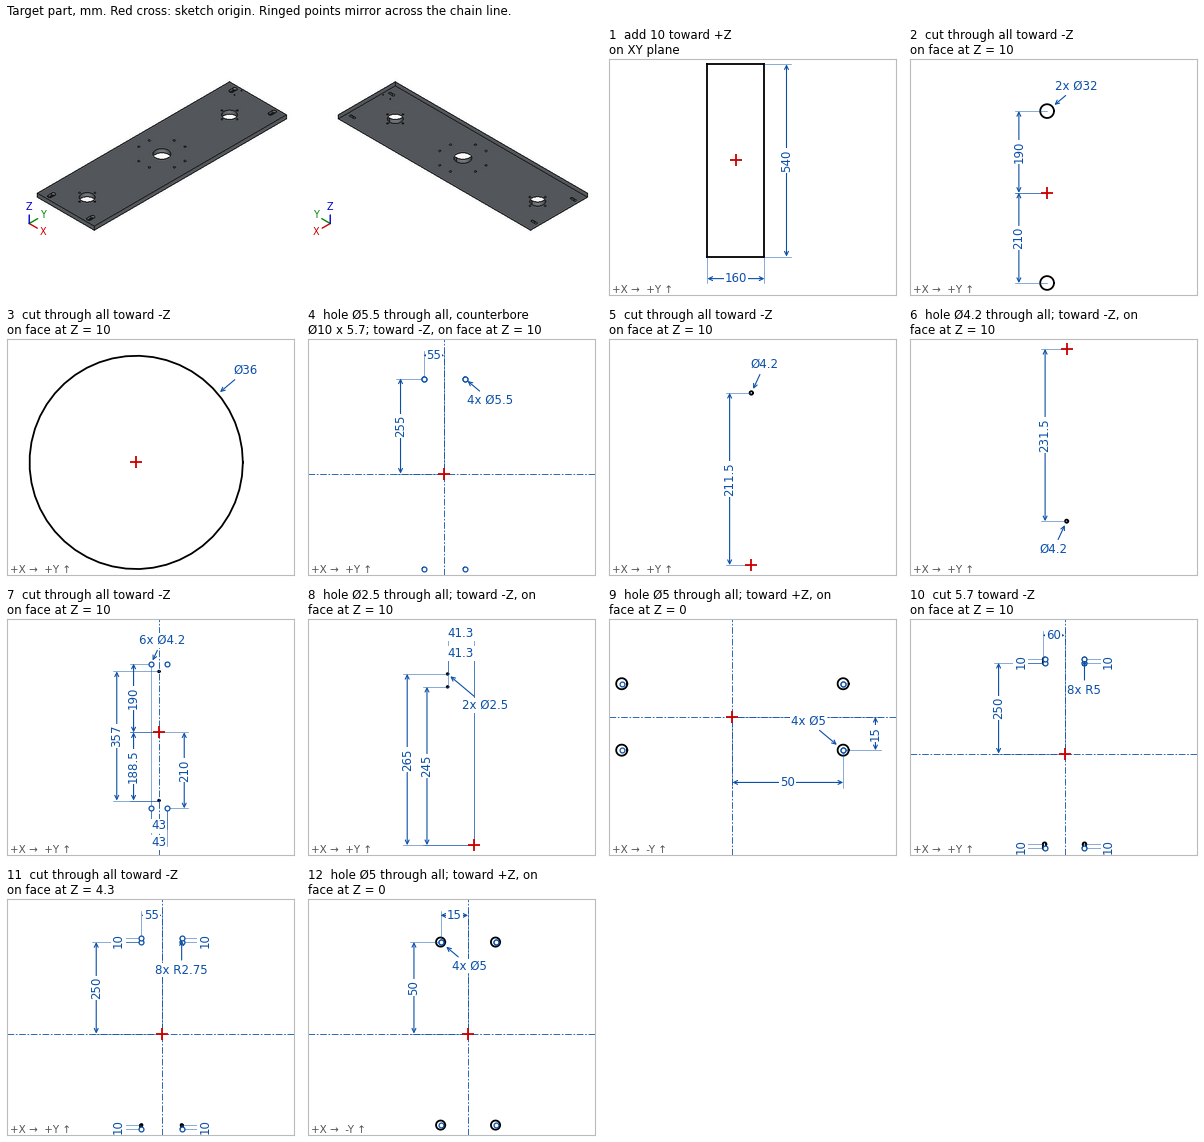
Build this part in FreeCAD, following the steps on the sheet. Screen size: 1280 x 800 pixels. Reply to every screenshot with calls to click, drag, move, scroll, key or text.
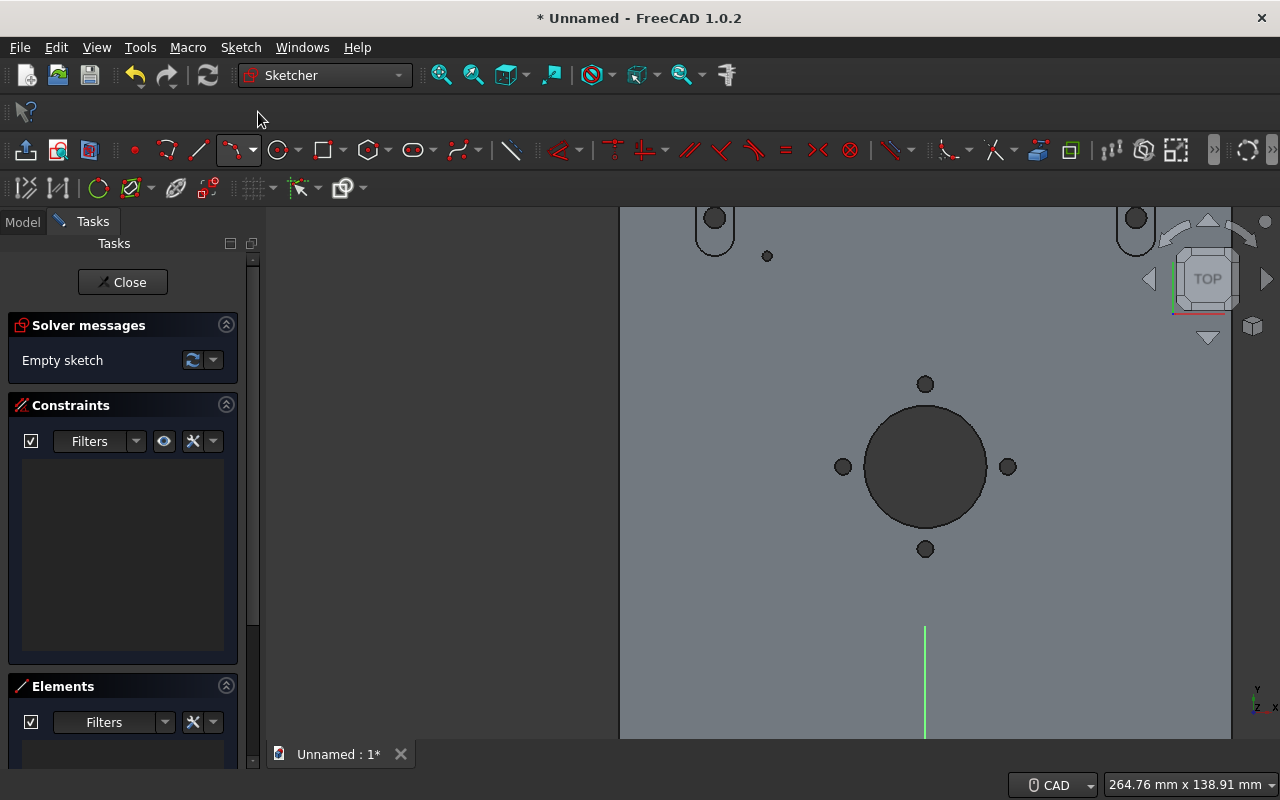
scroll(661, 330, down, 9)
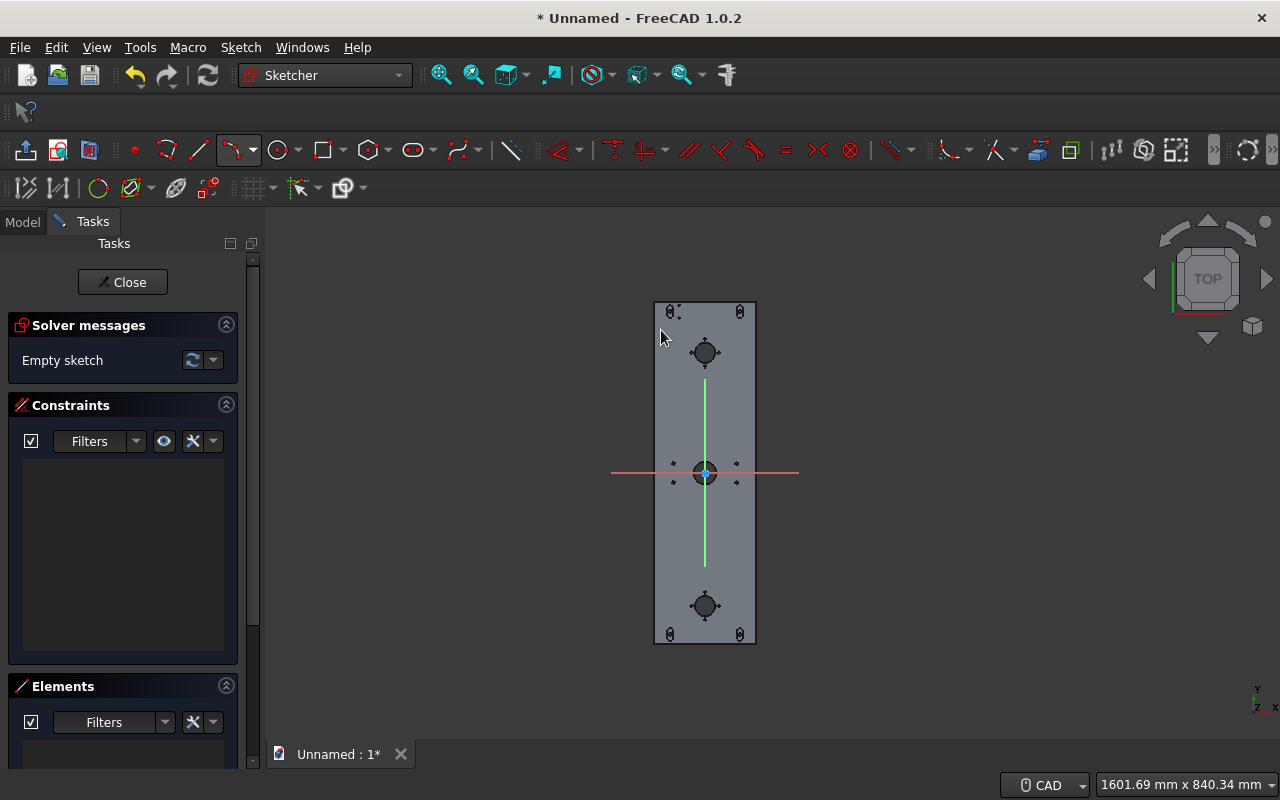
key(g)
key(s)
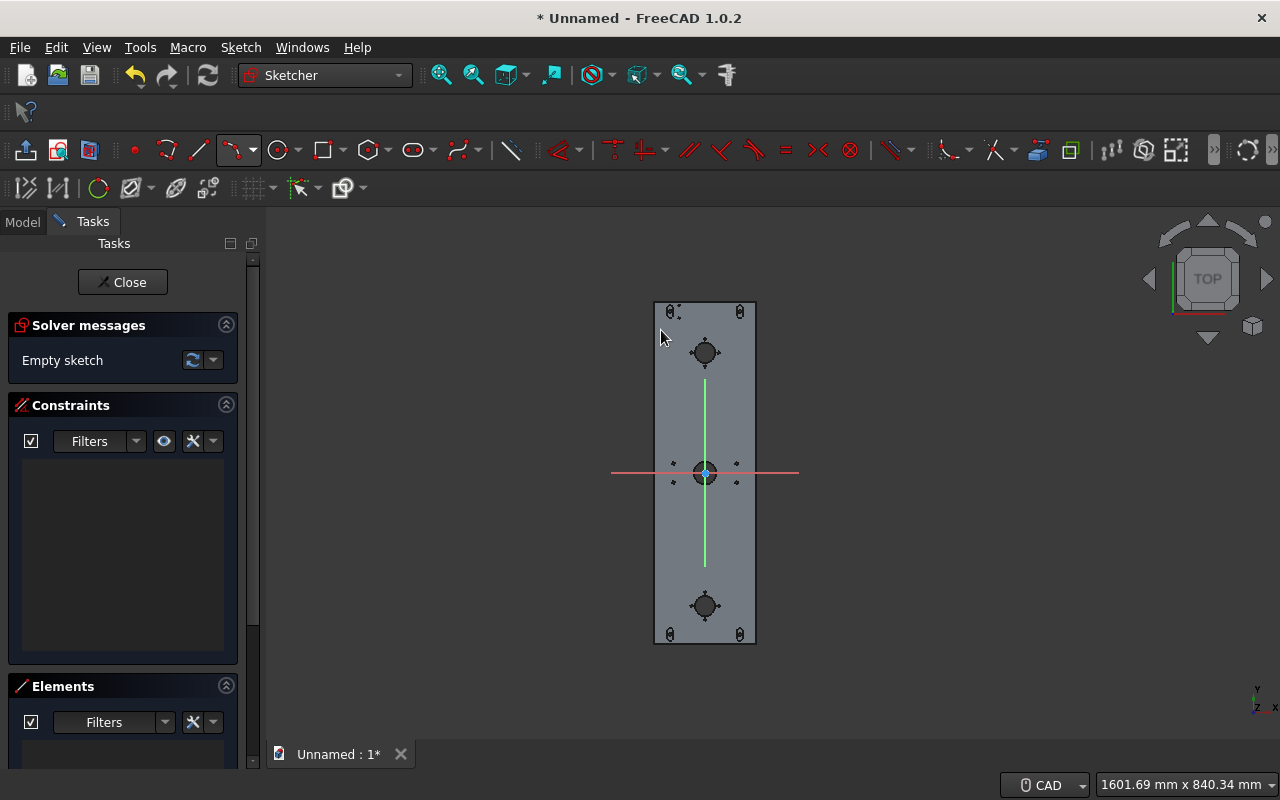
scroll(670, 315, up, 13)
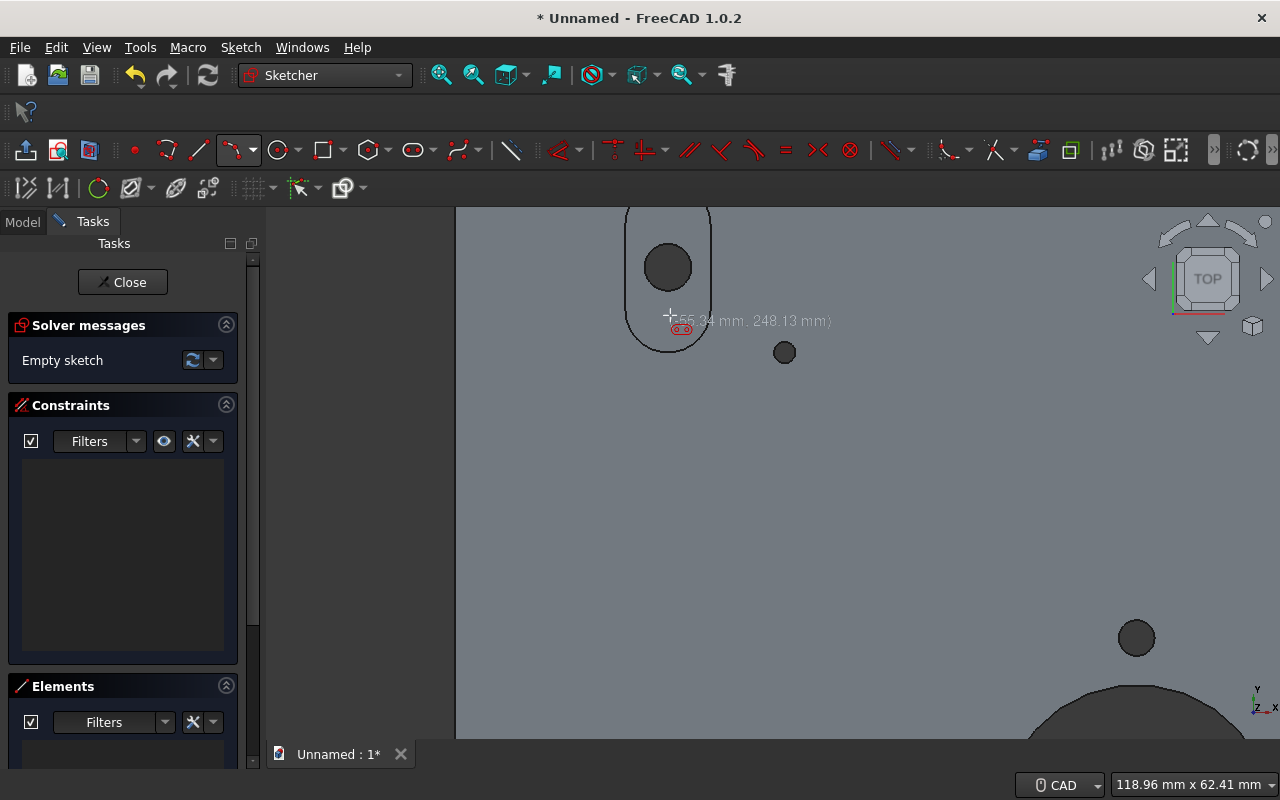
scroll(670, 315, down, 13)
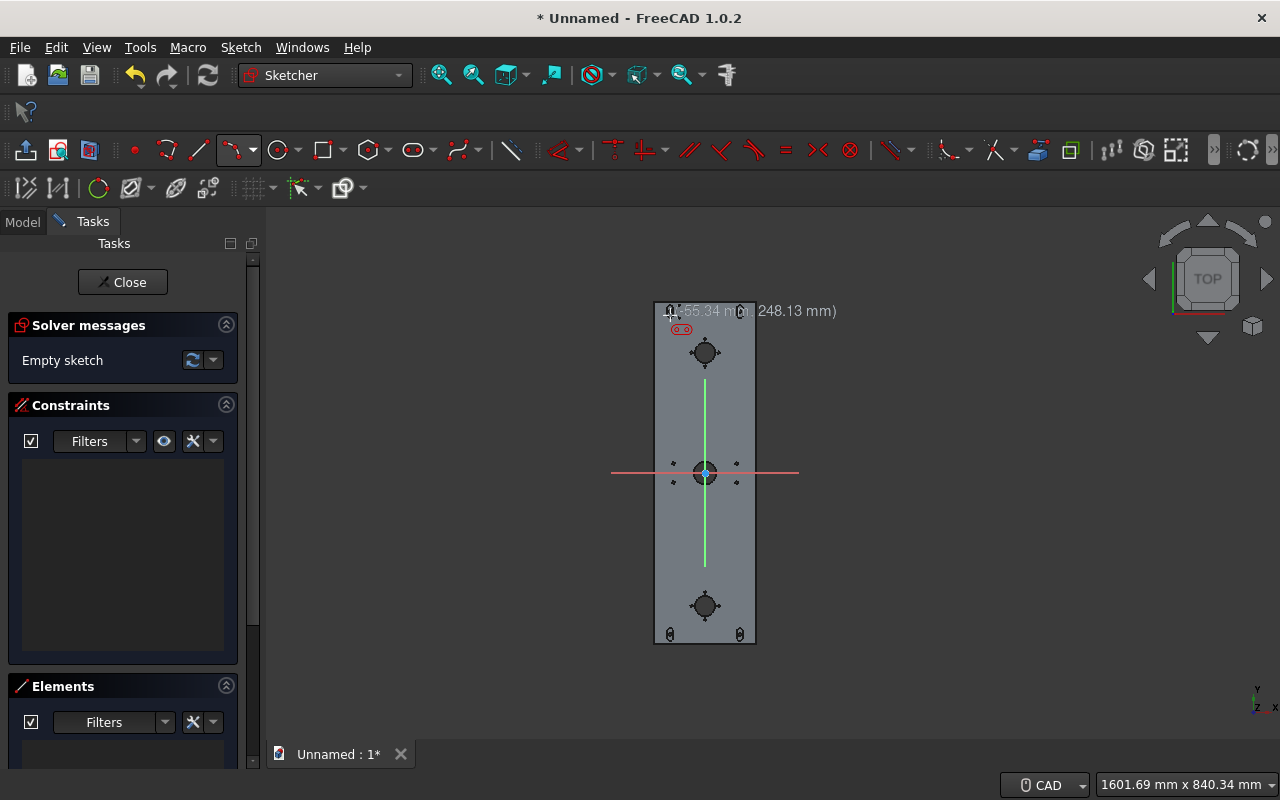
click(670, 315)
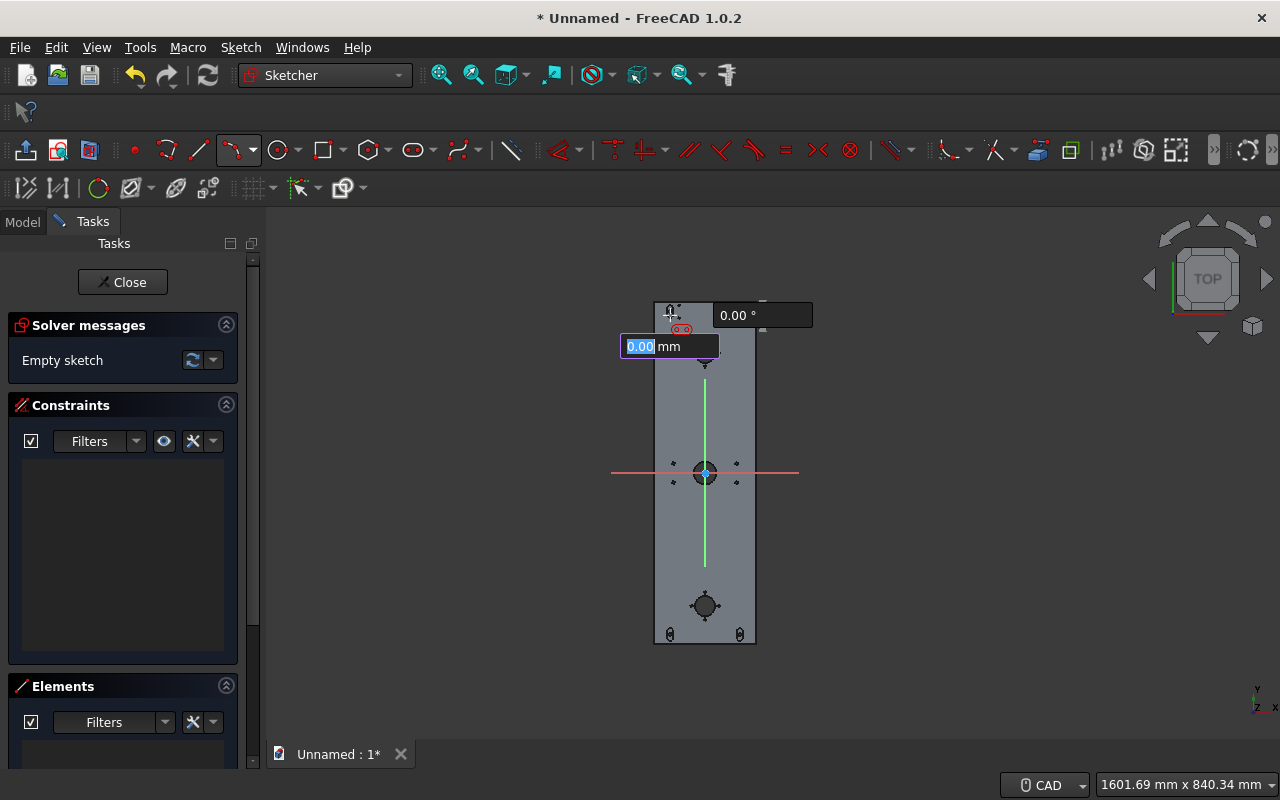
scroll(670, 308, up, 5)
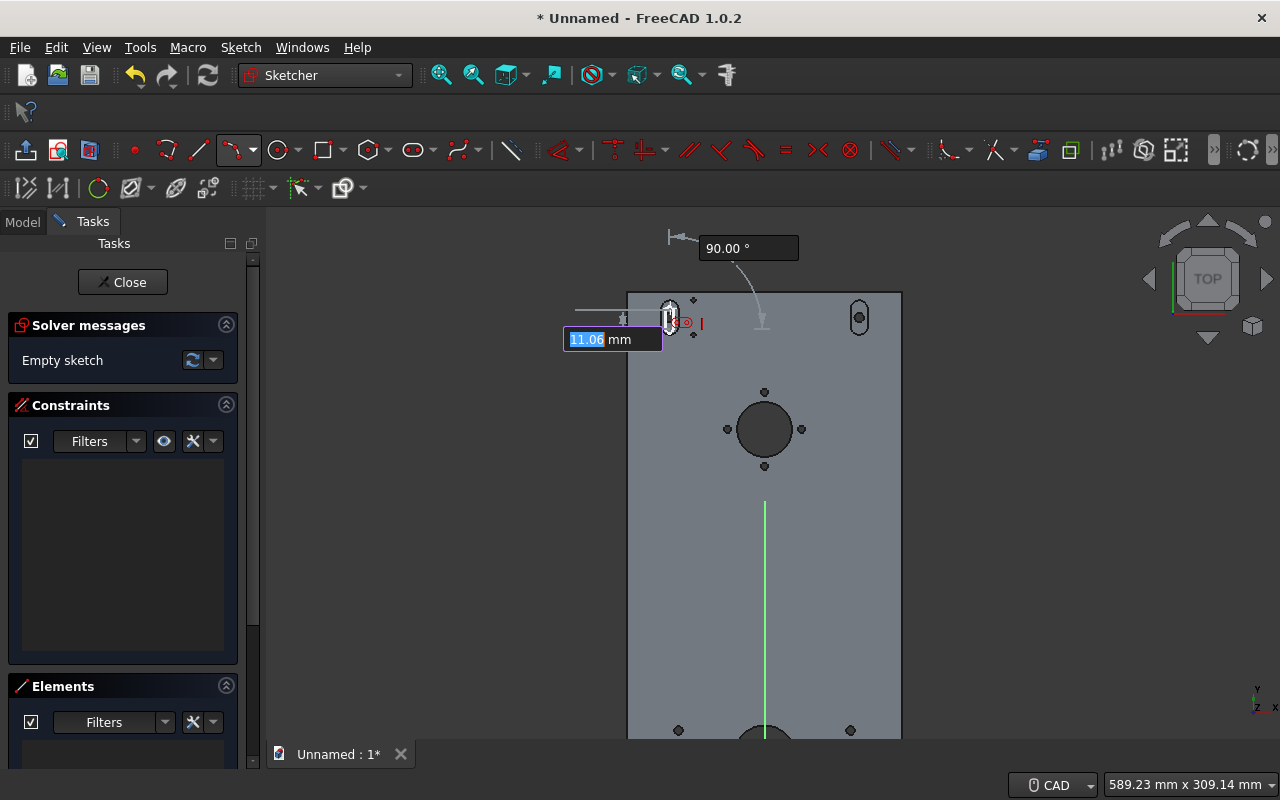
click(669, 309)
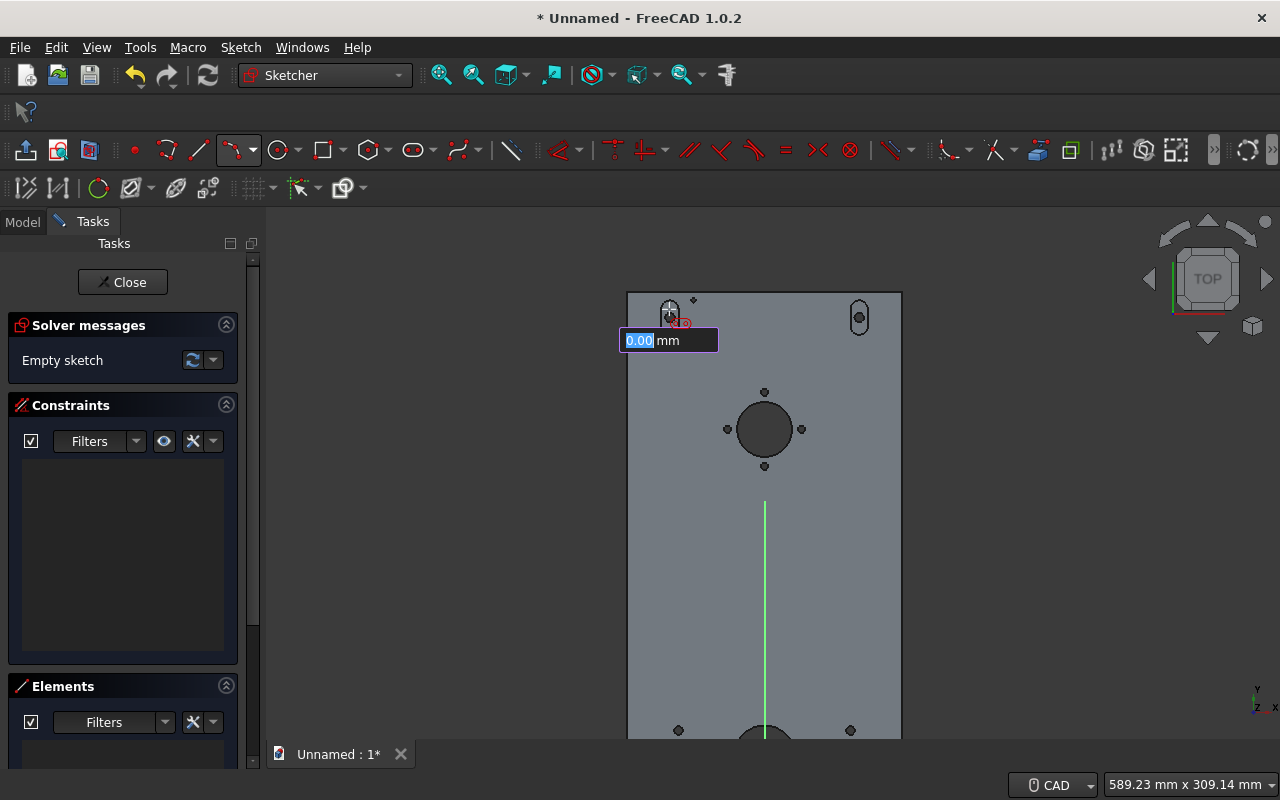
scroll(675, 318, up, 7)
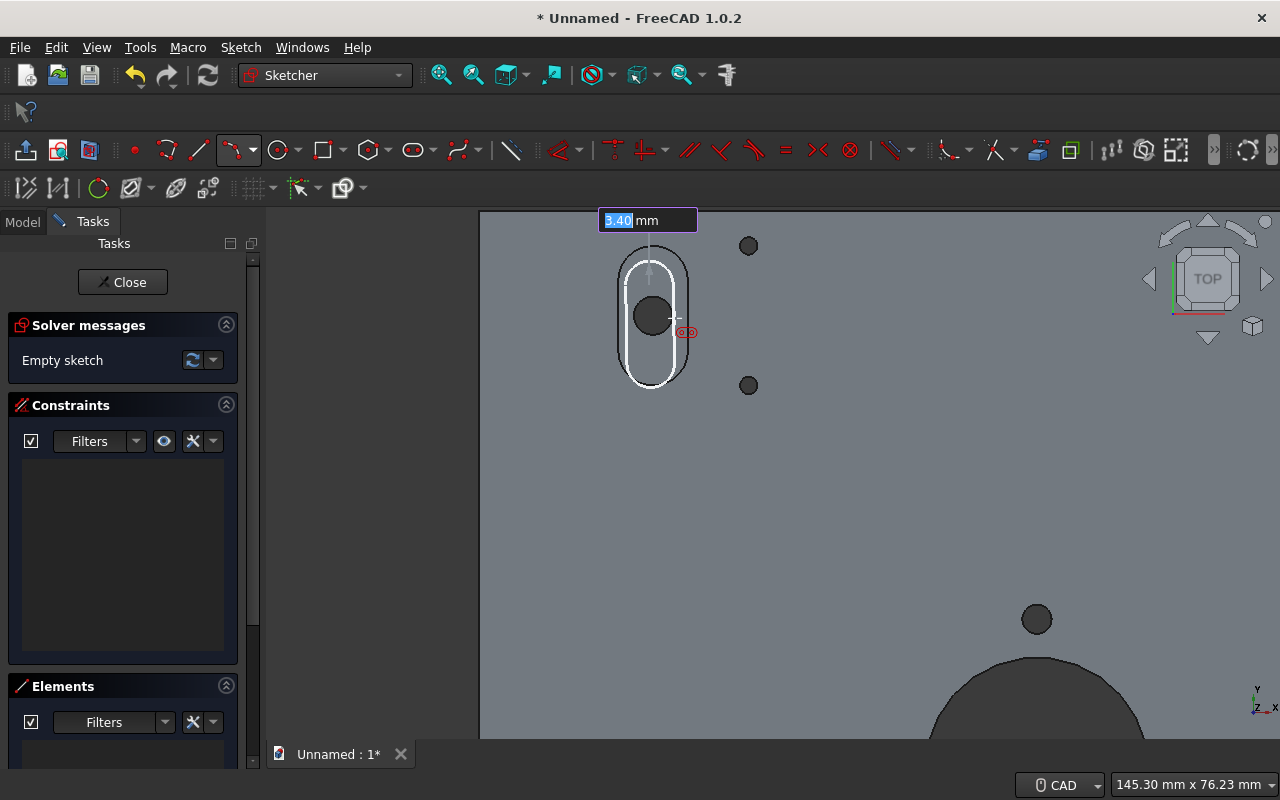
click(672, 316)